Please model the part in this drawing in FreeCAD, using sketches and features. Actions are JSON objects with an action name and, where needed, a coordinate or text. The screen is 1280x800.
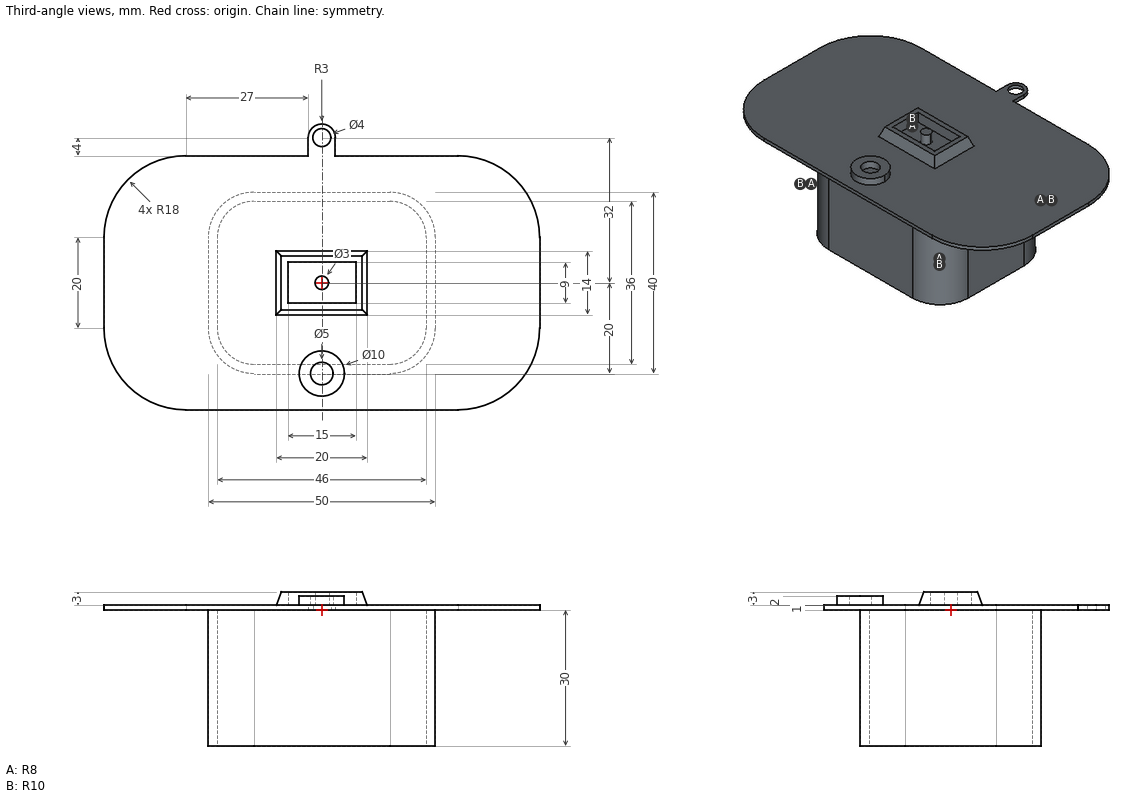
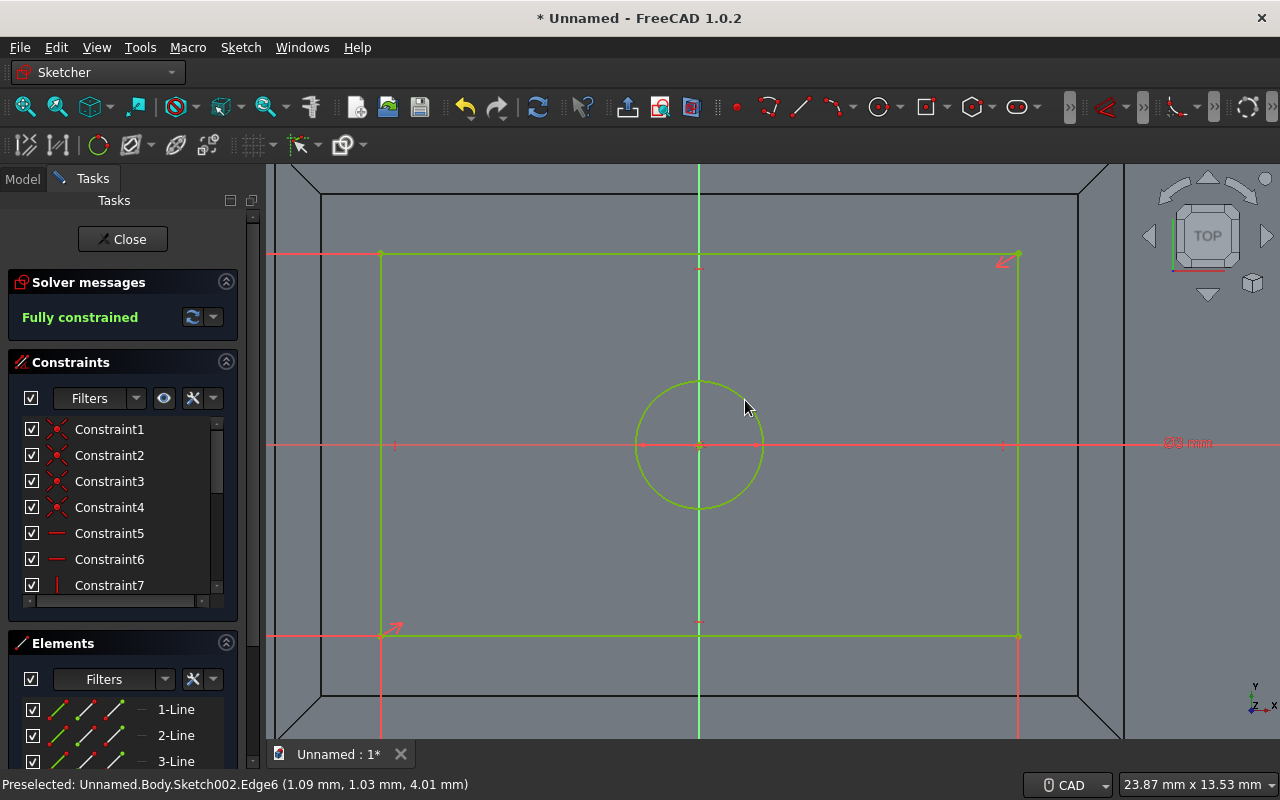
{"action": "left_click", "coordinate": [123, 239]}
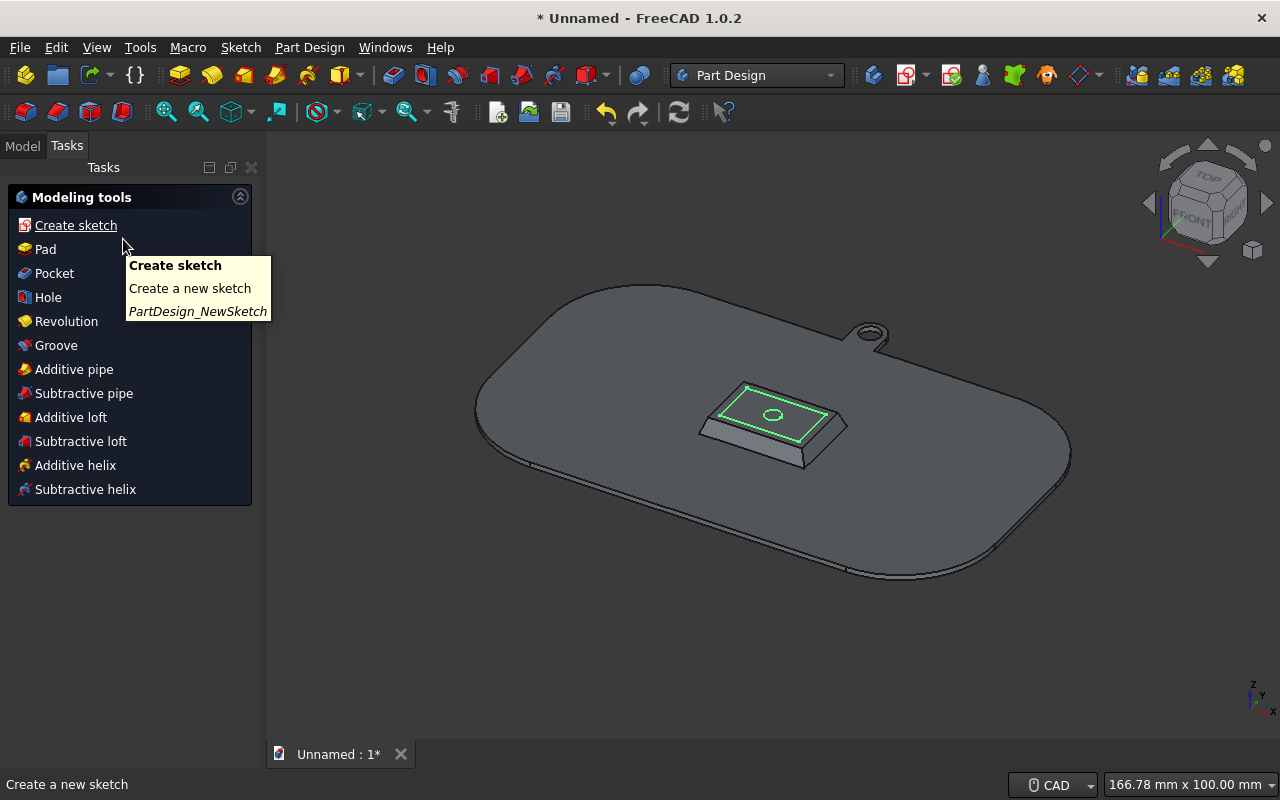
{"action": "left_click", "coordinate": [394, 76]}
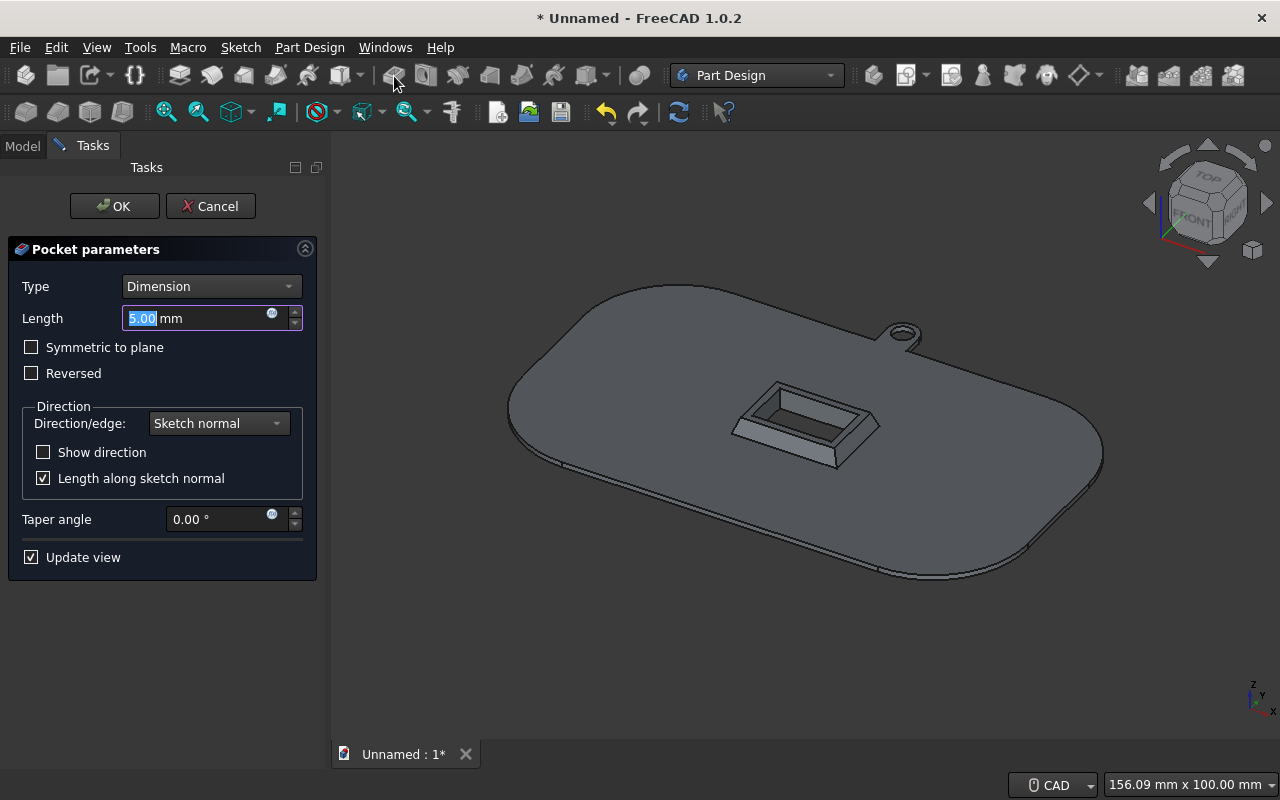
{"action": "type", "text": "3"}
{"action": "key", "text": "Tab"}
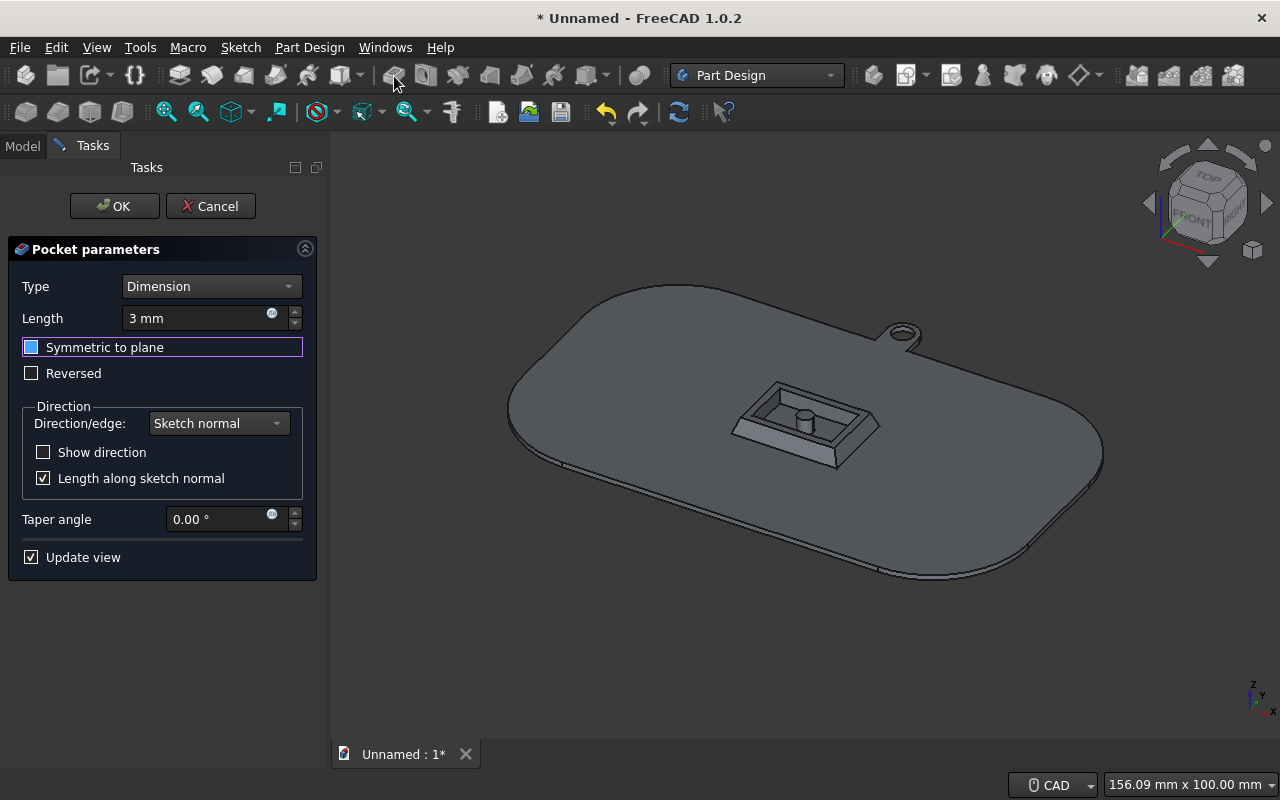
{"action": "left_click", "coordinate": [115, 206]}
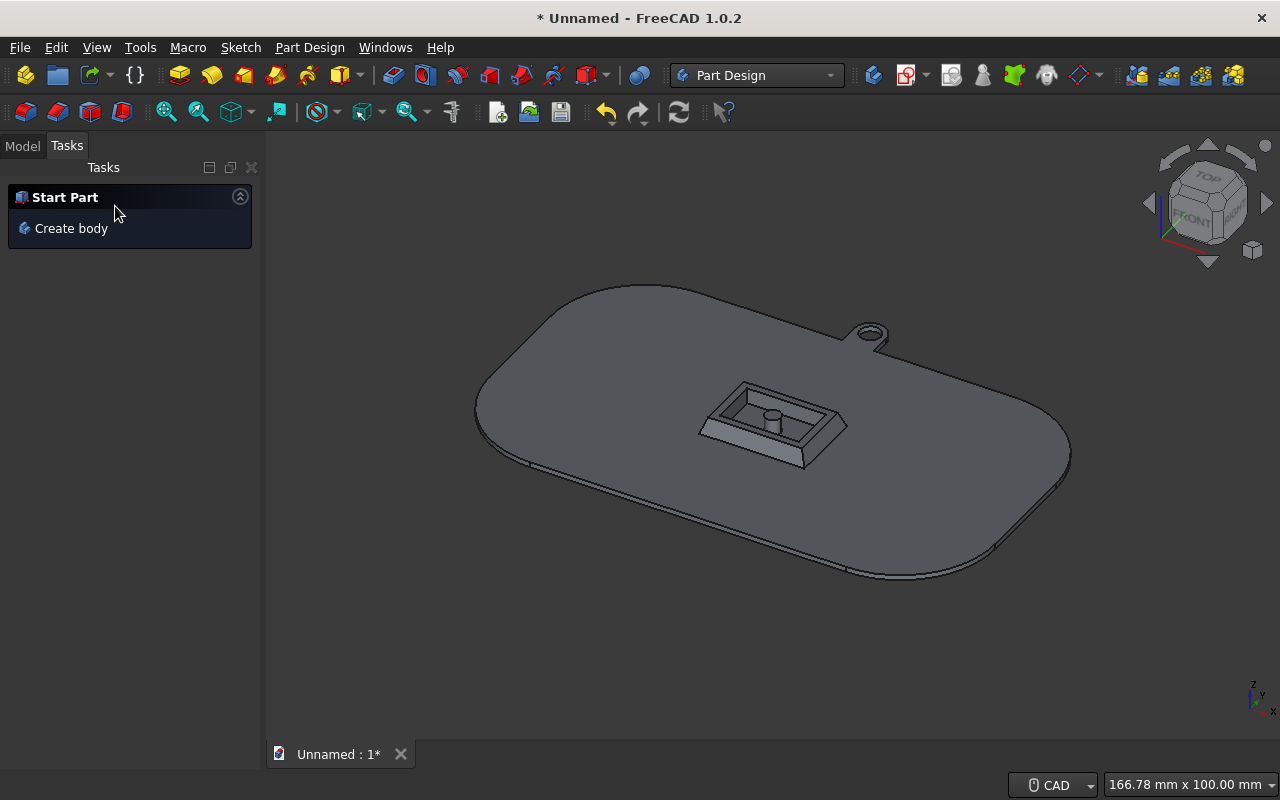
{"action": "left_click", "coordinate": [906, 76]}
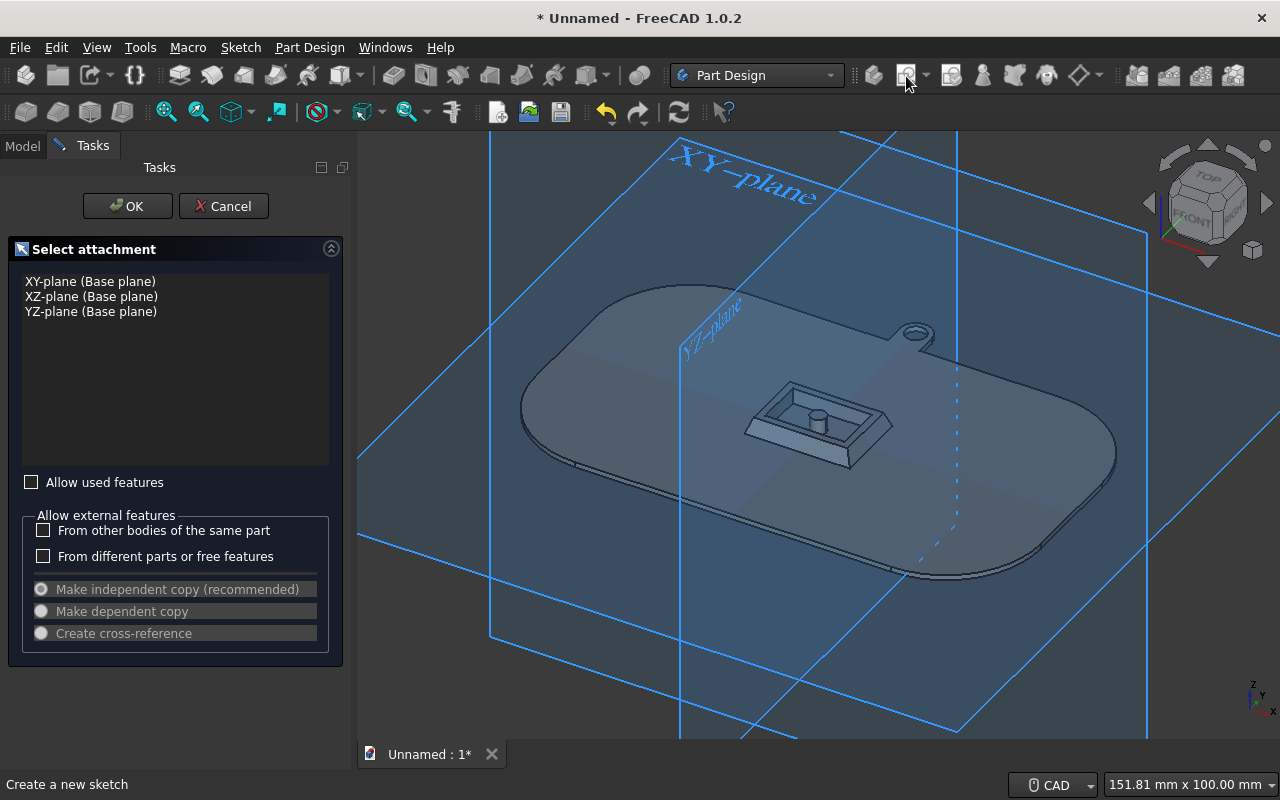
{"action": "left_click", "coordinate": [82, 282]}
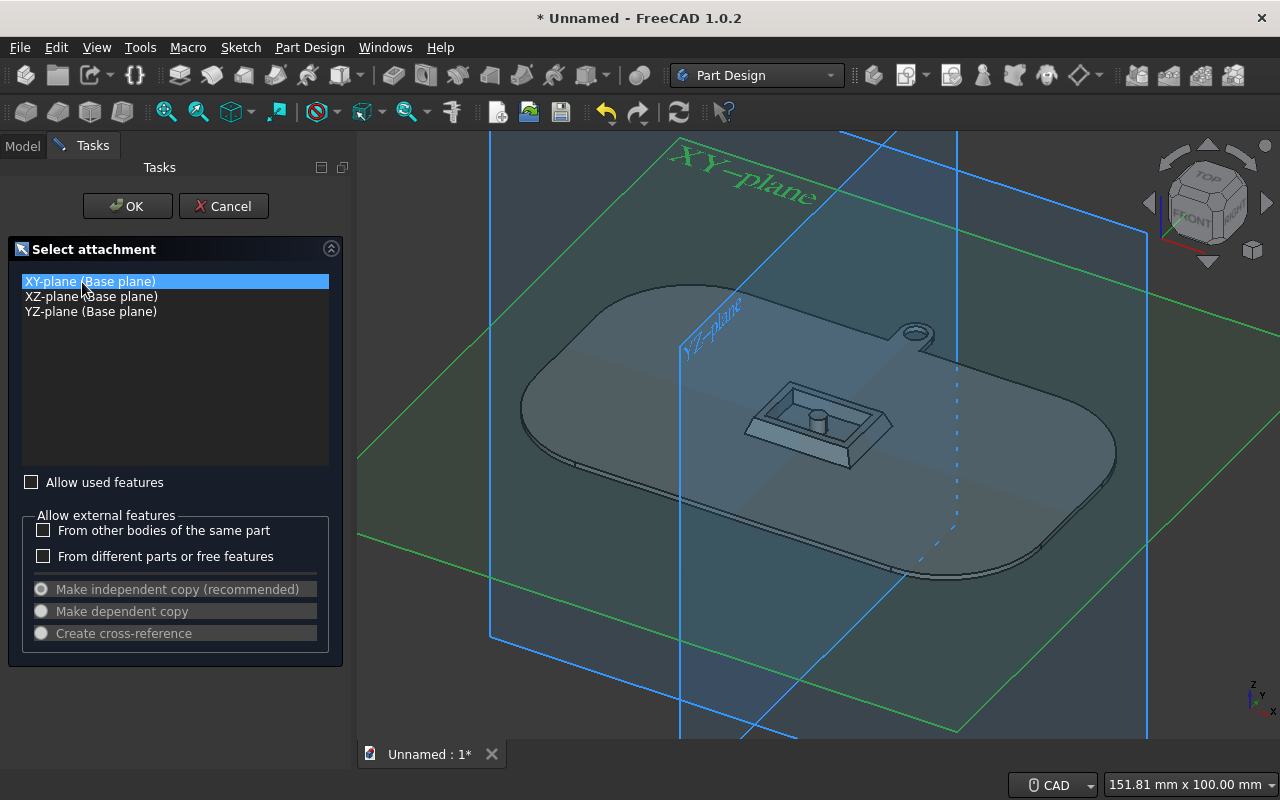
{"action": "left_click", "coordinate": [128, 206]}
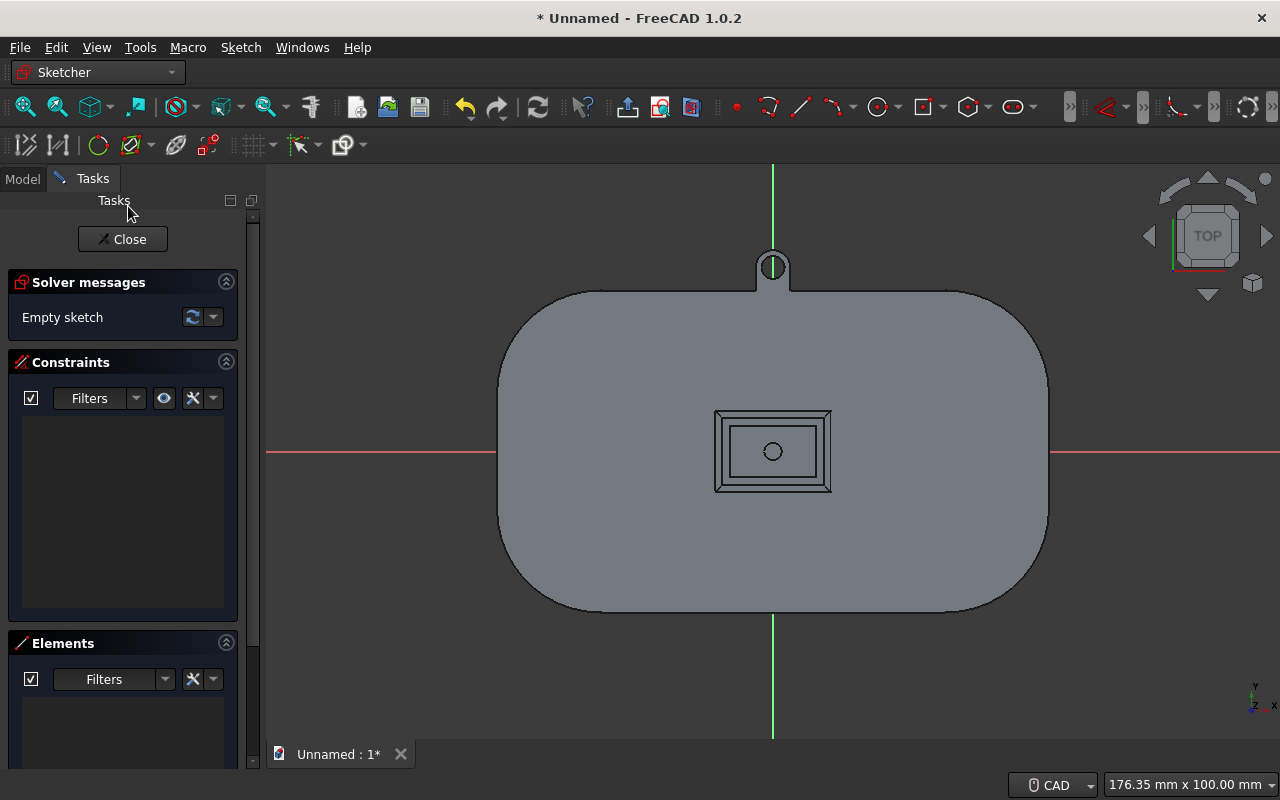
{"action": "left_click", "coordinate": [692, 108]}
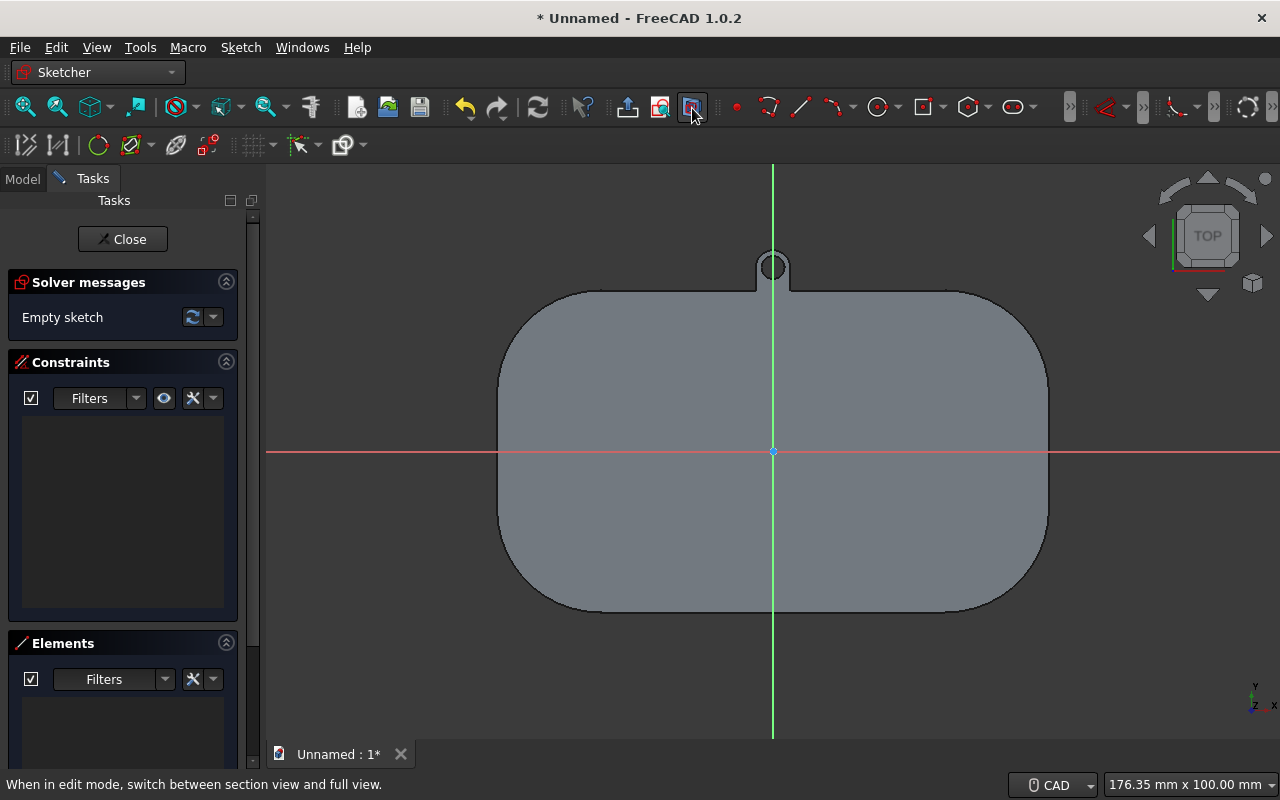
{"action": "scroll", "coordinate": [912, 452], "scroll_direction": "up", "scroll_amount": 2}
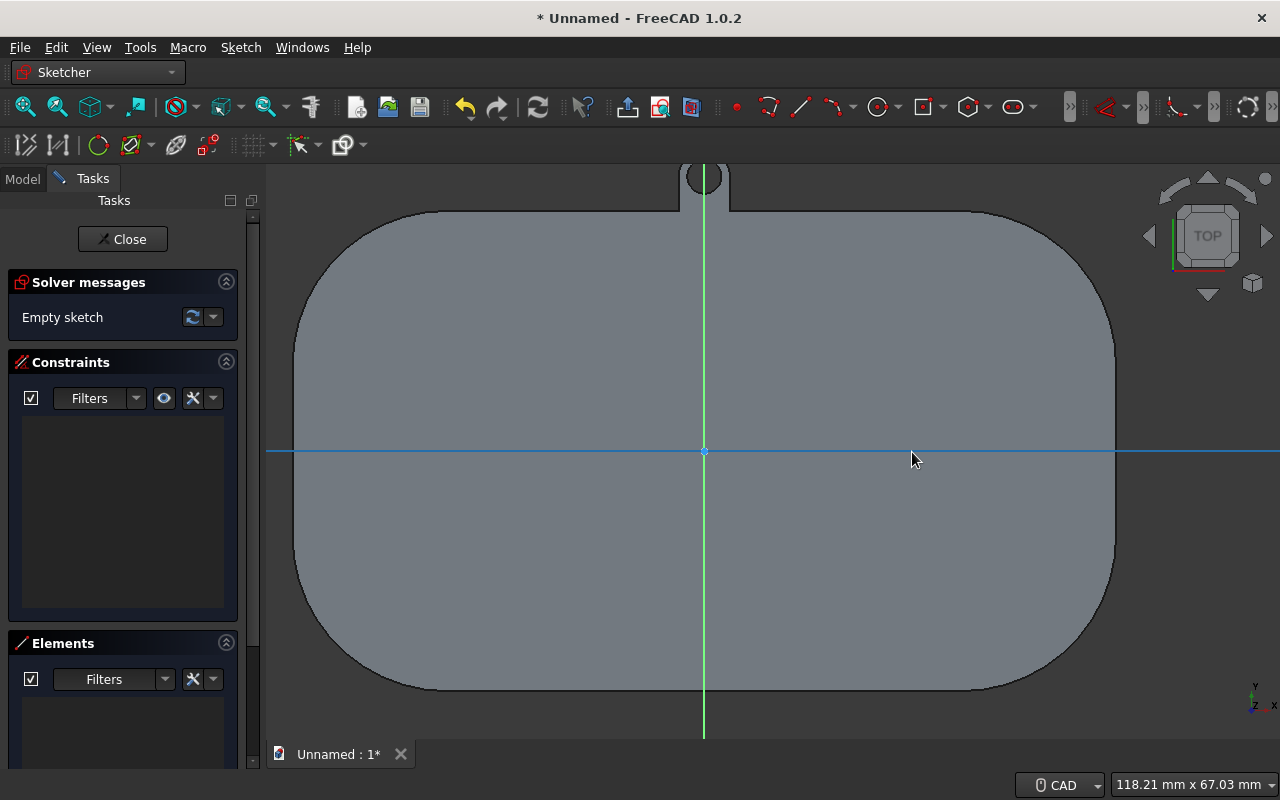
{"action": "left_click", "coordinate": [924, 108]}